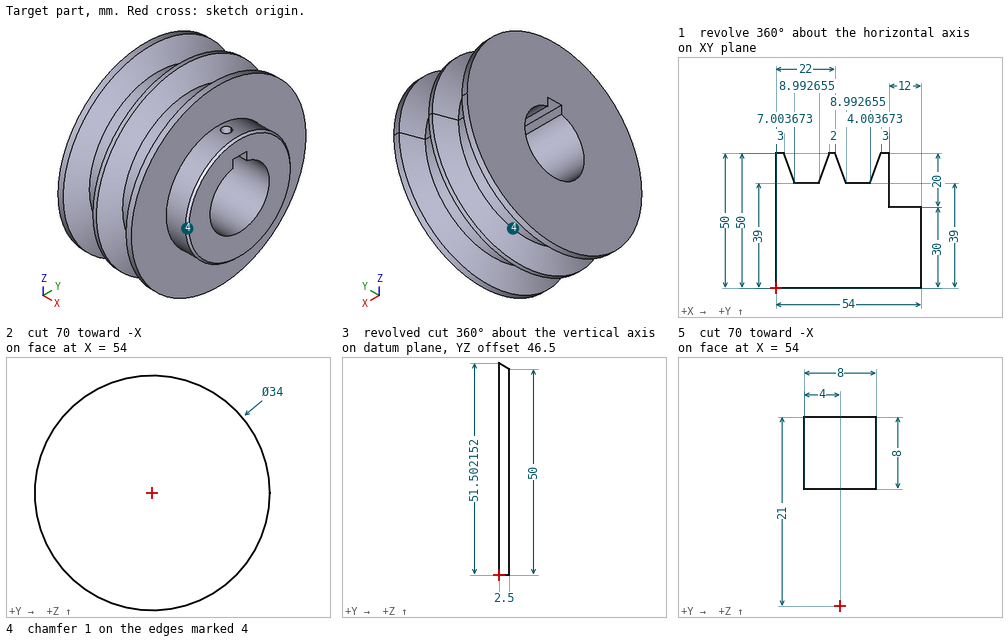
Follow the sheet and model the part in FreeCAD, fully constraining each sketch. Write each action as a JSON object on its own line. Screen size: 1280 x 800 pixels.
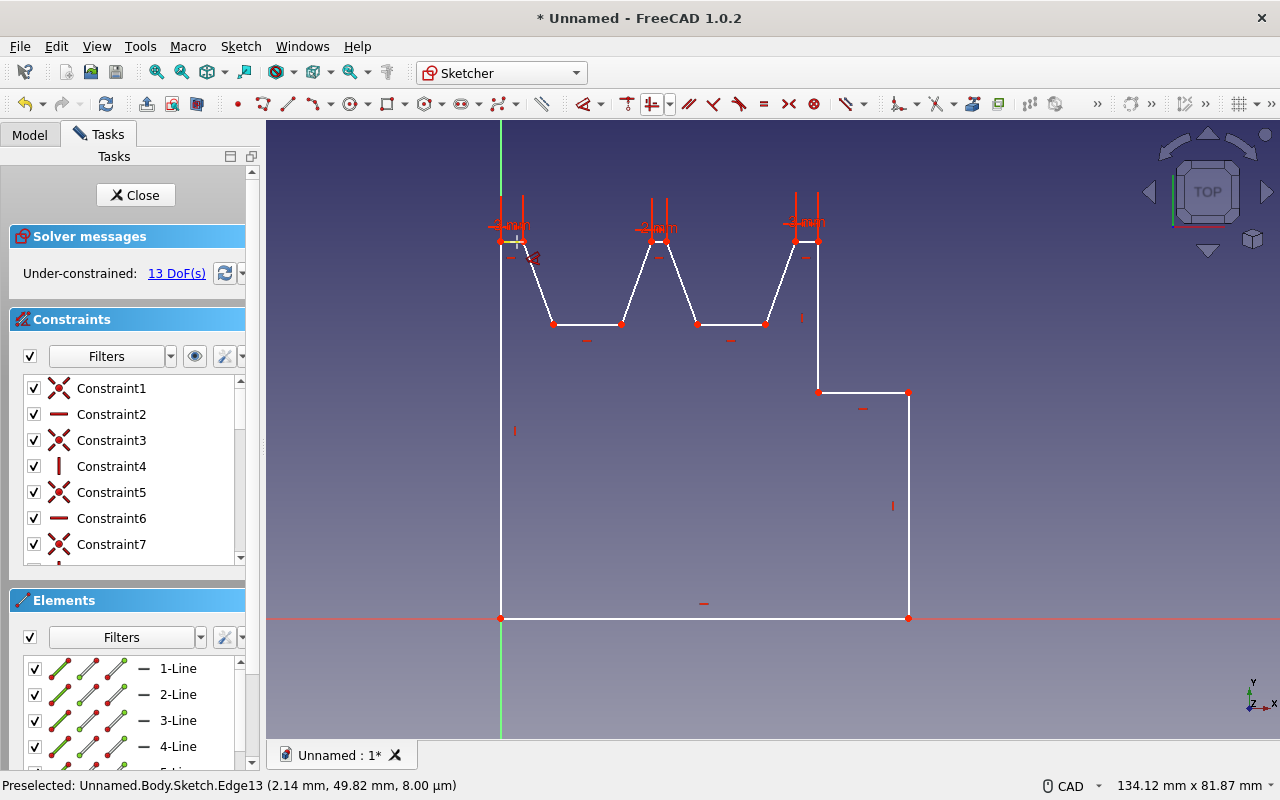
{"action": "left_click", "coordinate": [623, 619]}
{"action": "left_click", "coordinate": [705, 653]}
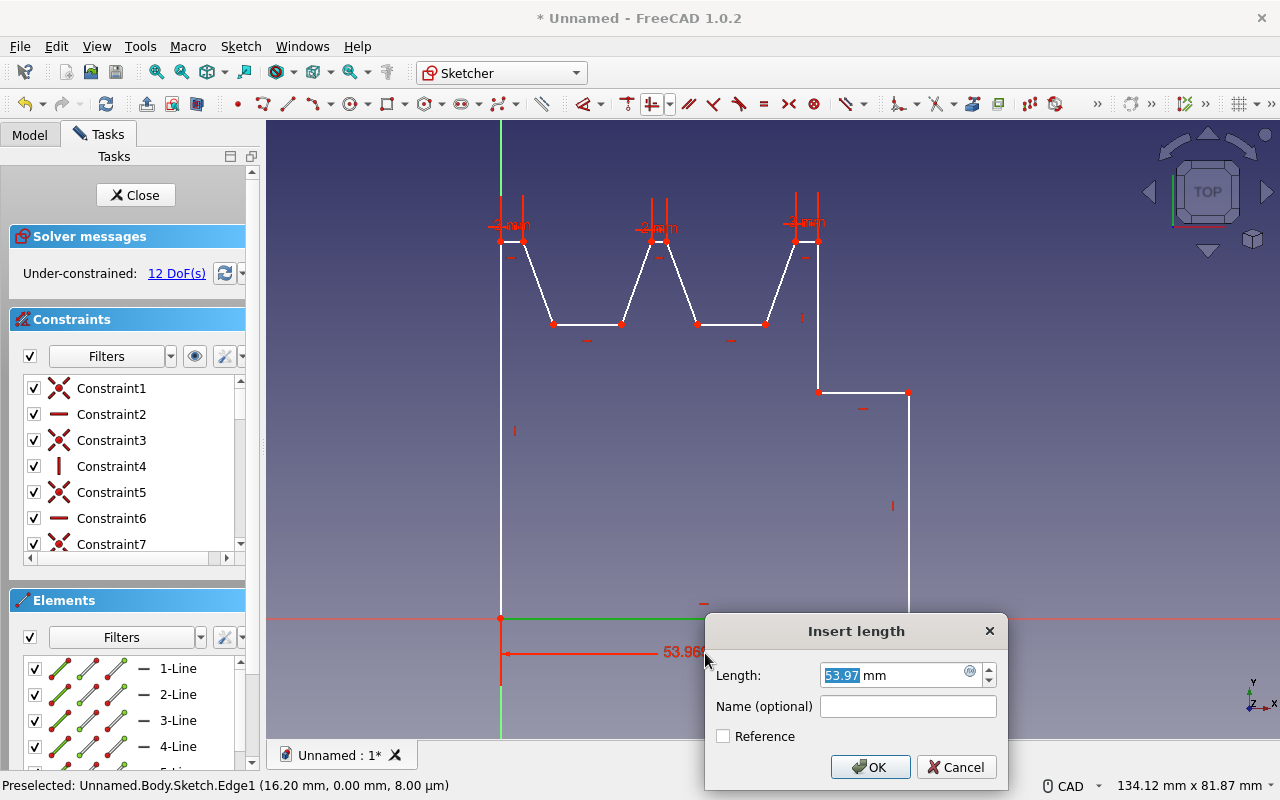
{"action": "type", "text": "54"}
{"action": "key", "text": "Return"}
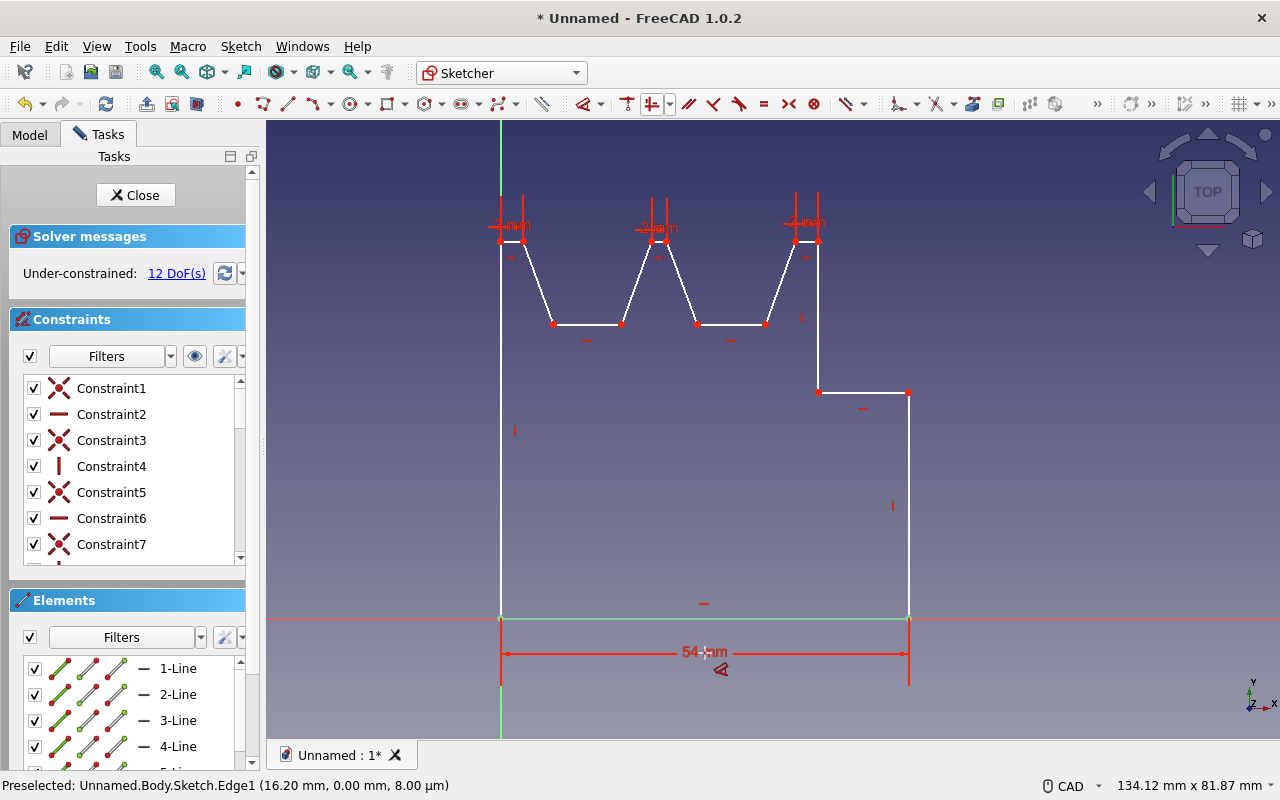
{"action": "left_click", "coordinate": [909, 551]}
{"action": "left_click", "coordinate": [943, 506]}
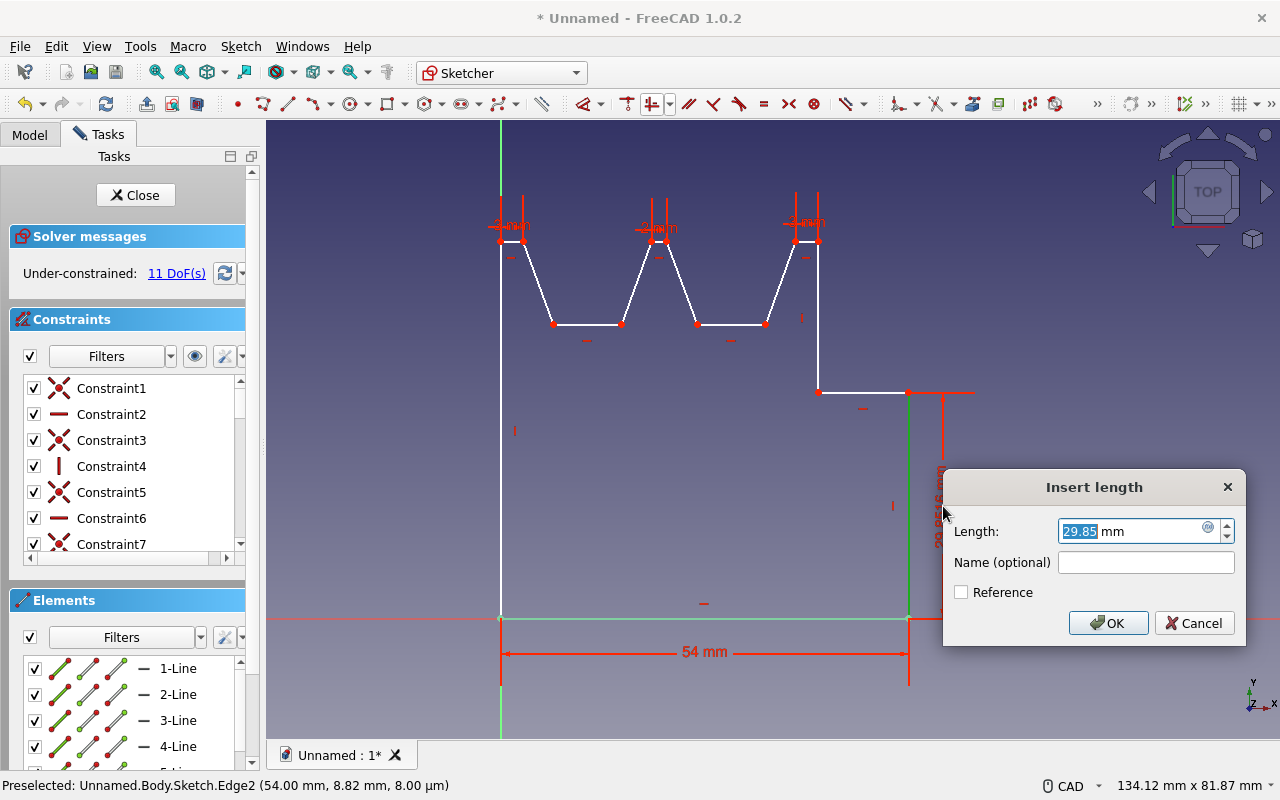
{"action": "type", "text": "30"}
{"action": "key", "text": "Return"}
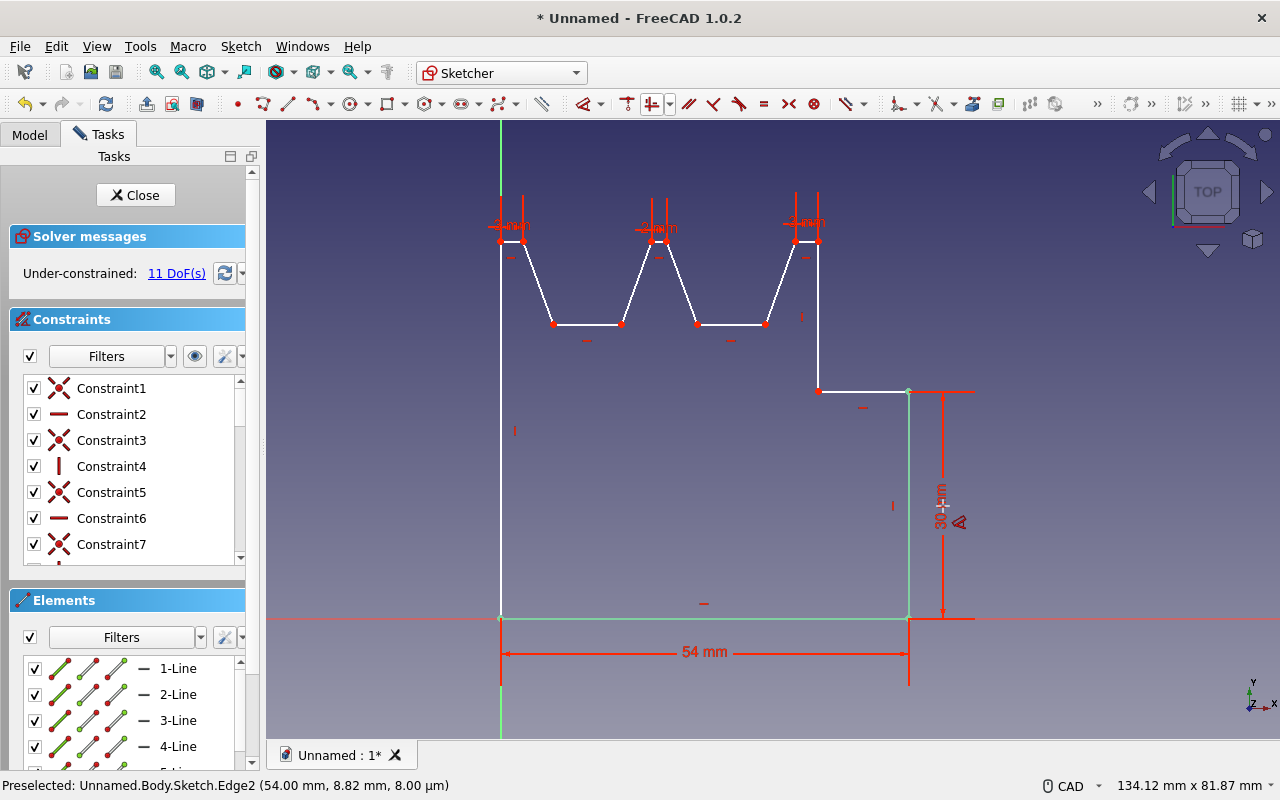
{"action": "left_click", "coordinate": [882, 392]}
{"action": "left_click", "coordinate": [863, 358]}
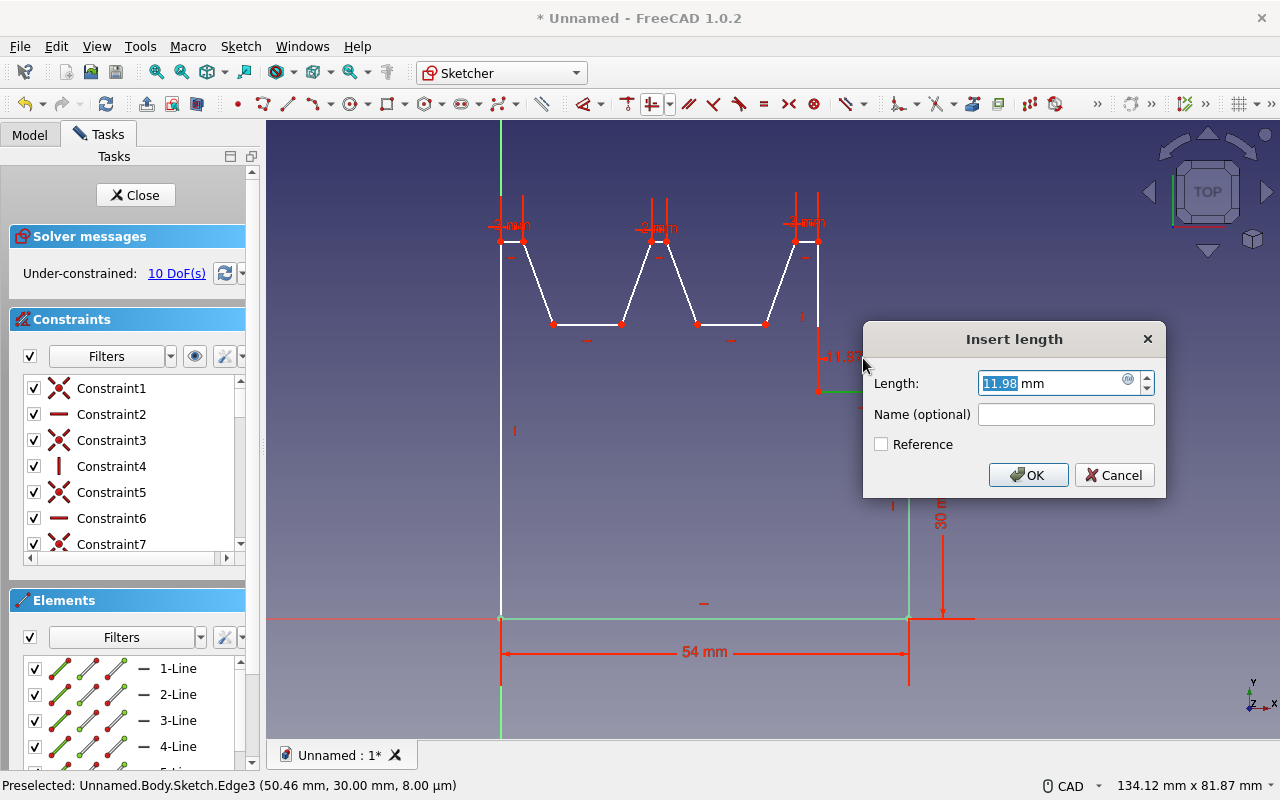
{"action": "type", "text": "12"}
{"action": "key", "text": "Return"}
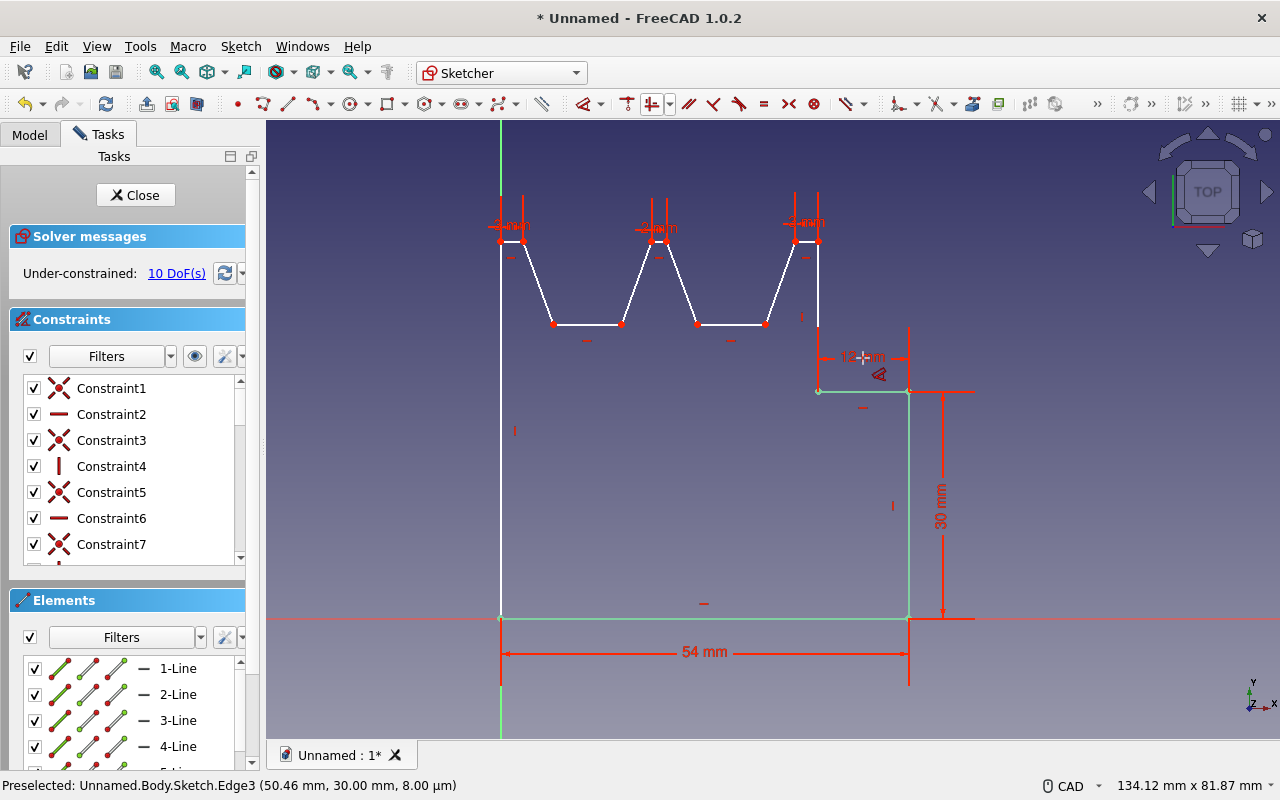
{"action": "left_click", "coordinate": [818, 347]}
{"action": "left_click", "coordinate": [852, 317]}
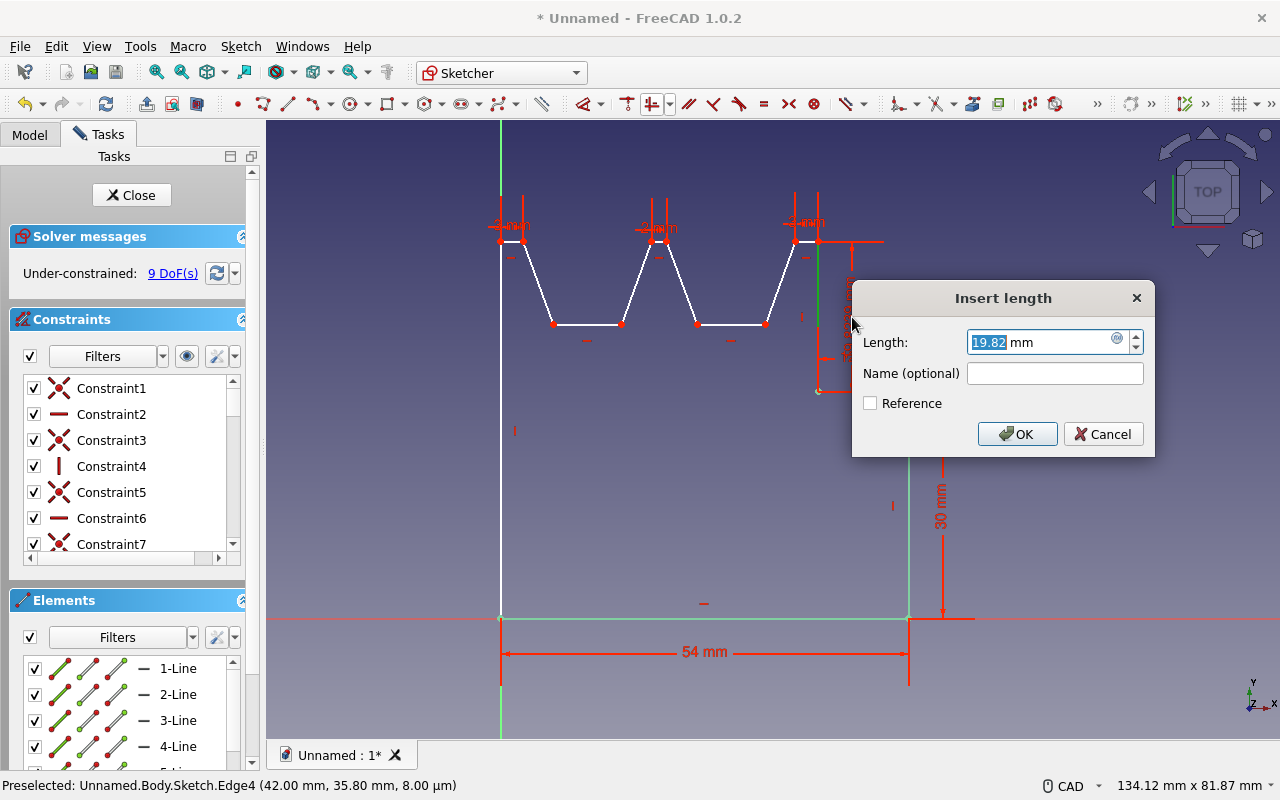
{"action": "type", "text": "20"}
{"action": "key", "text": "Return"}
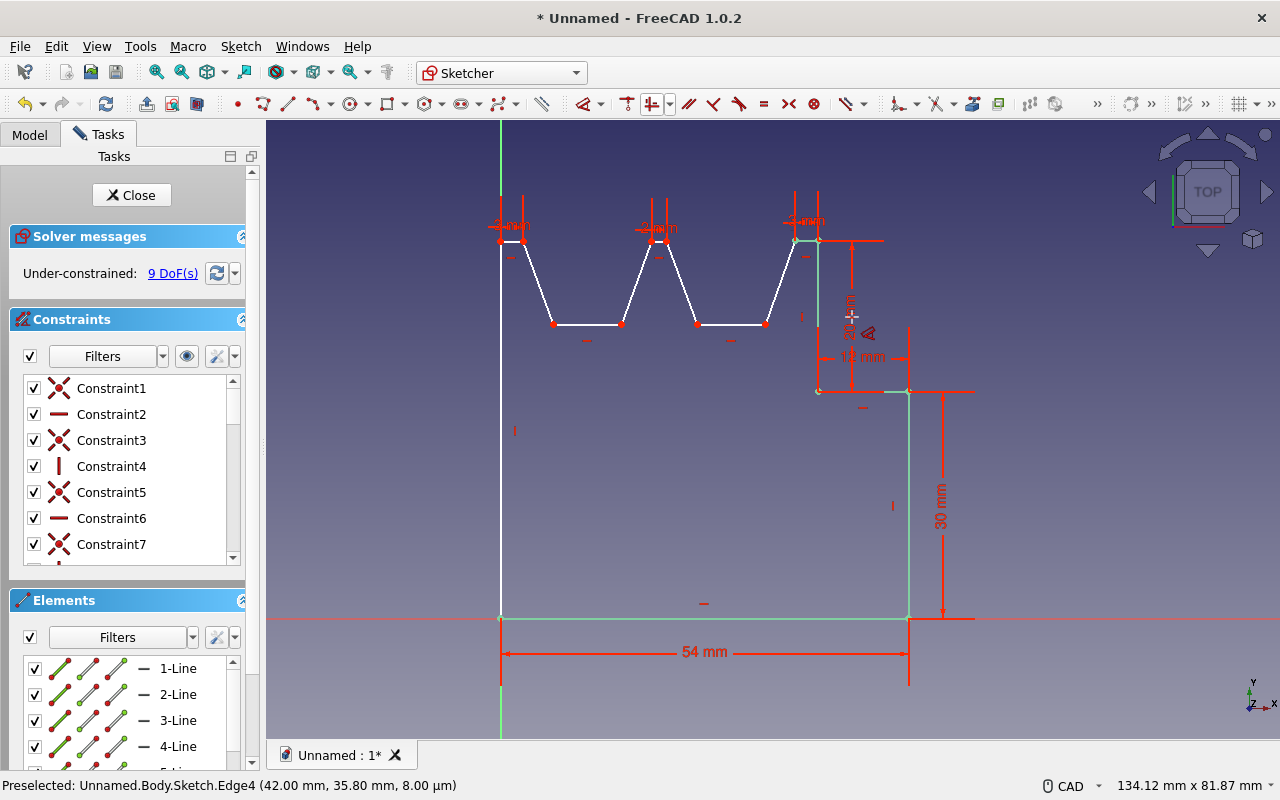
{"action": "left_click", "coordinate": [501, 355]}
{"action": "left_click", "coordinate": [467, 430]}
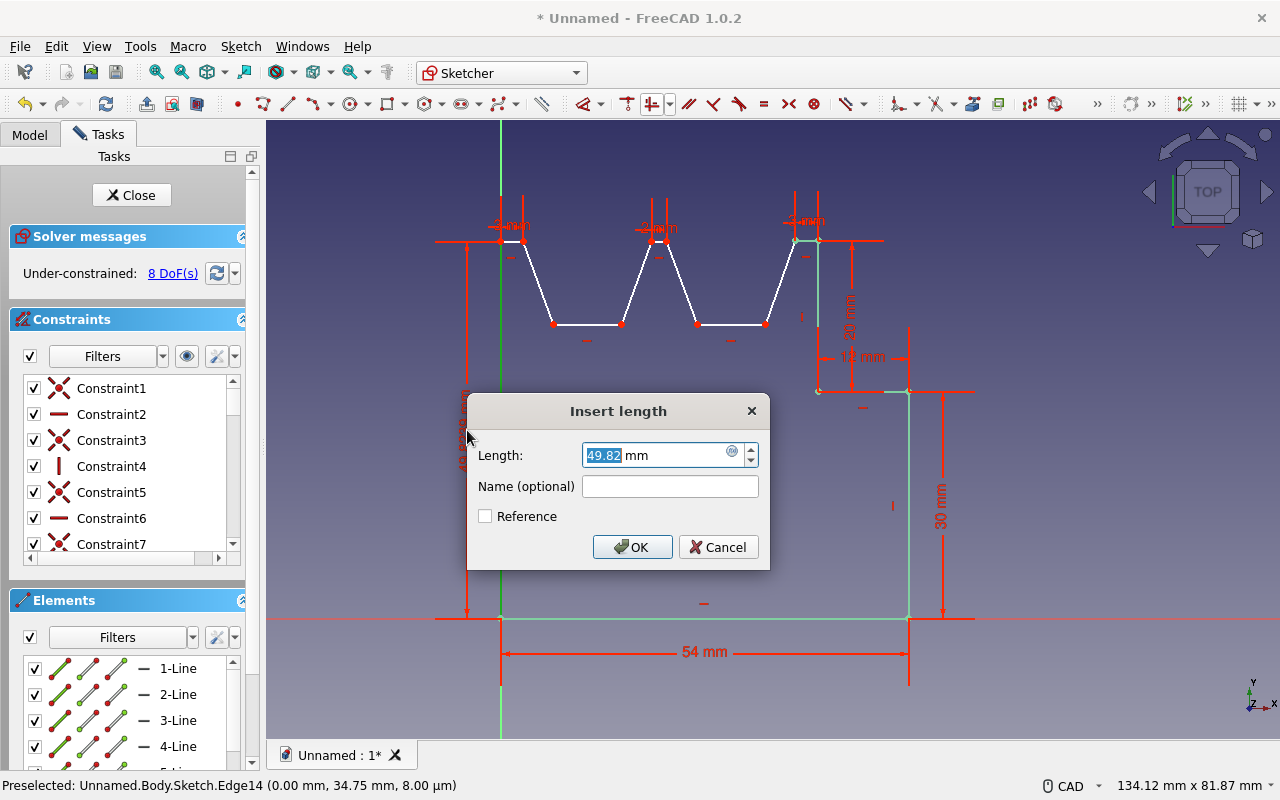
{"action": "type", "text": "50"}
{"action": "key", "text": "Return"}